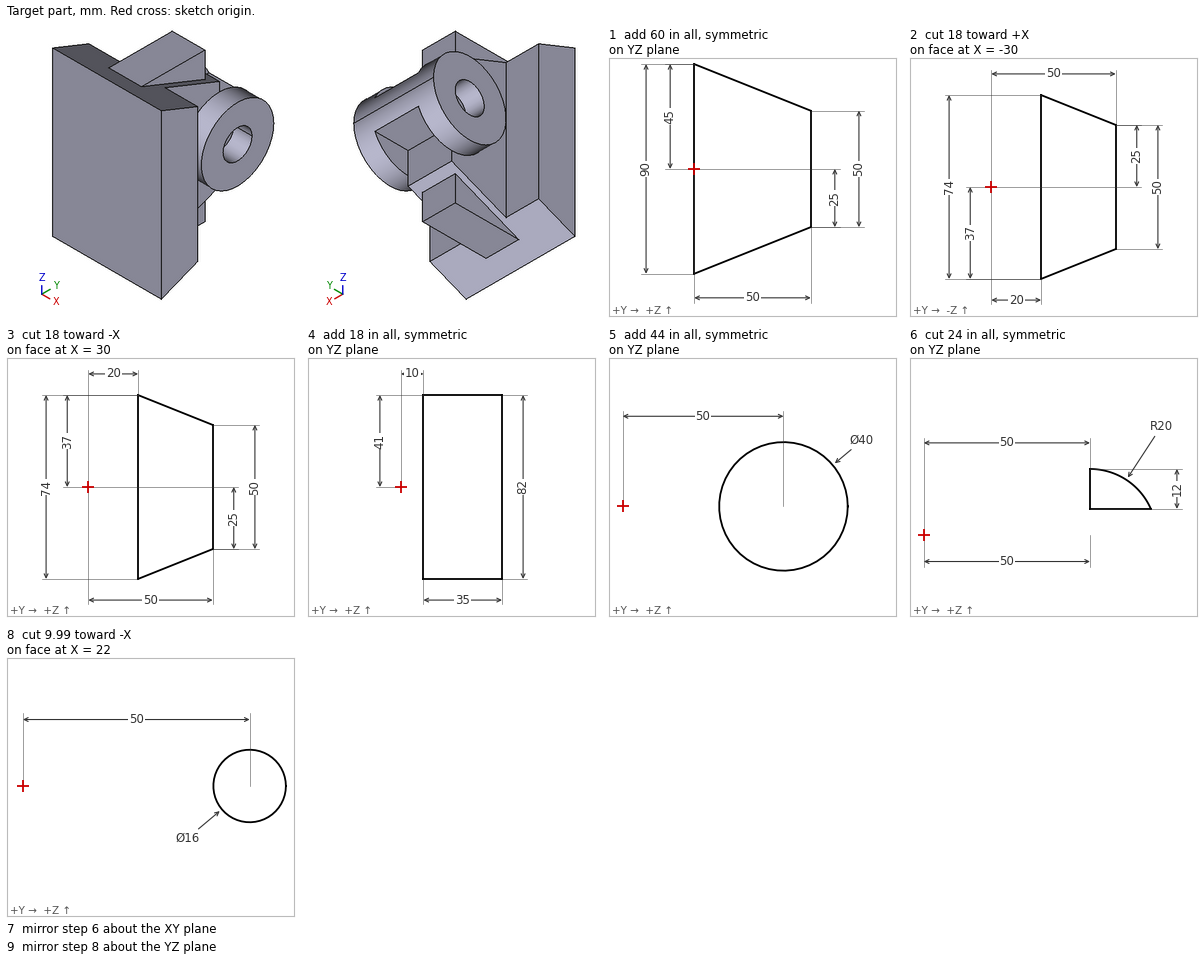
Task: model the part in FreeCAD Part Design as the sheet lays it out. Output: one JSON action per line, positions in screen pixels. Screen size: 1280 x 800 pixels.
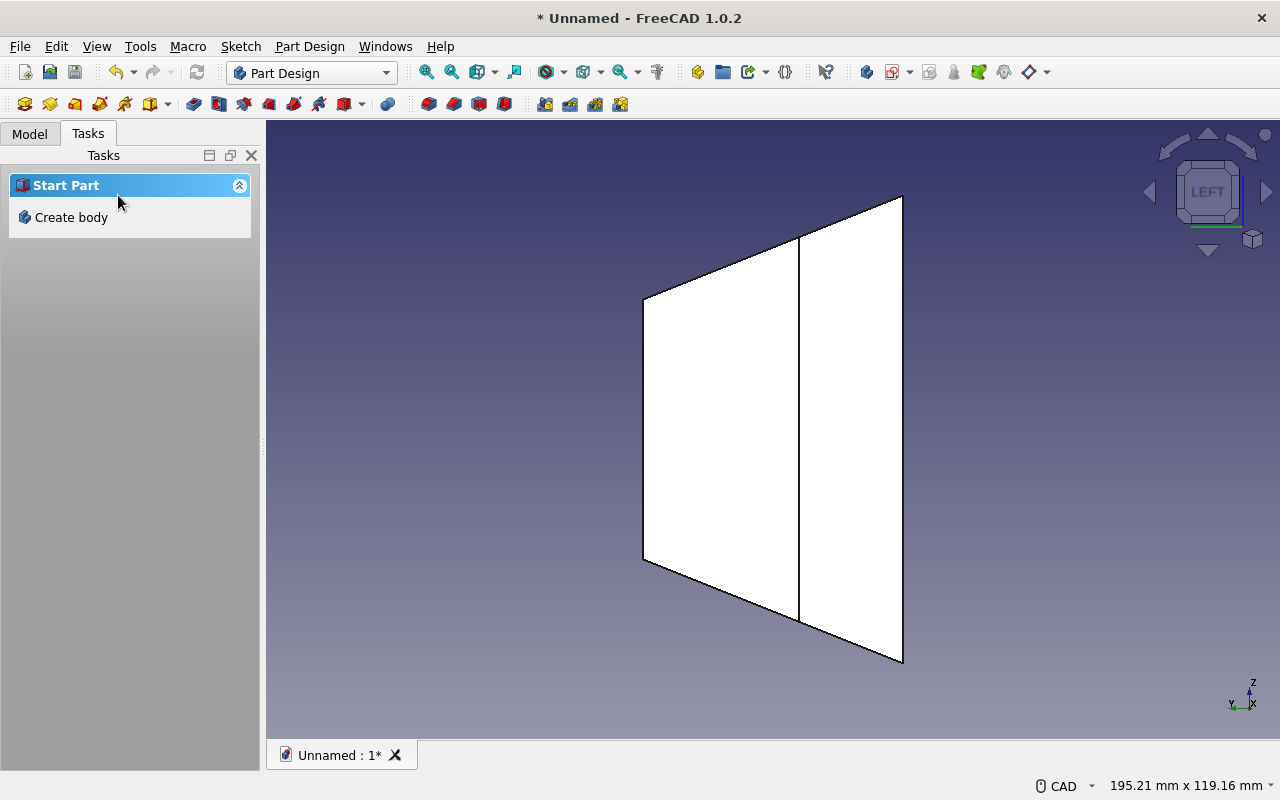
{"action": "key", "text": "0"}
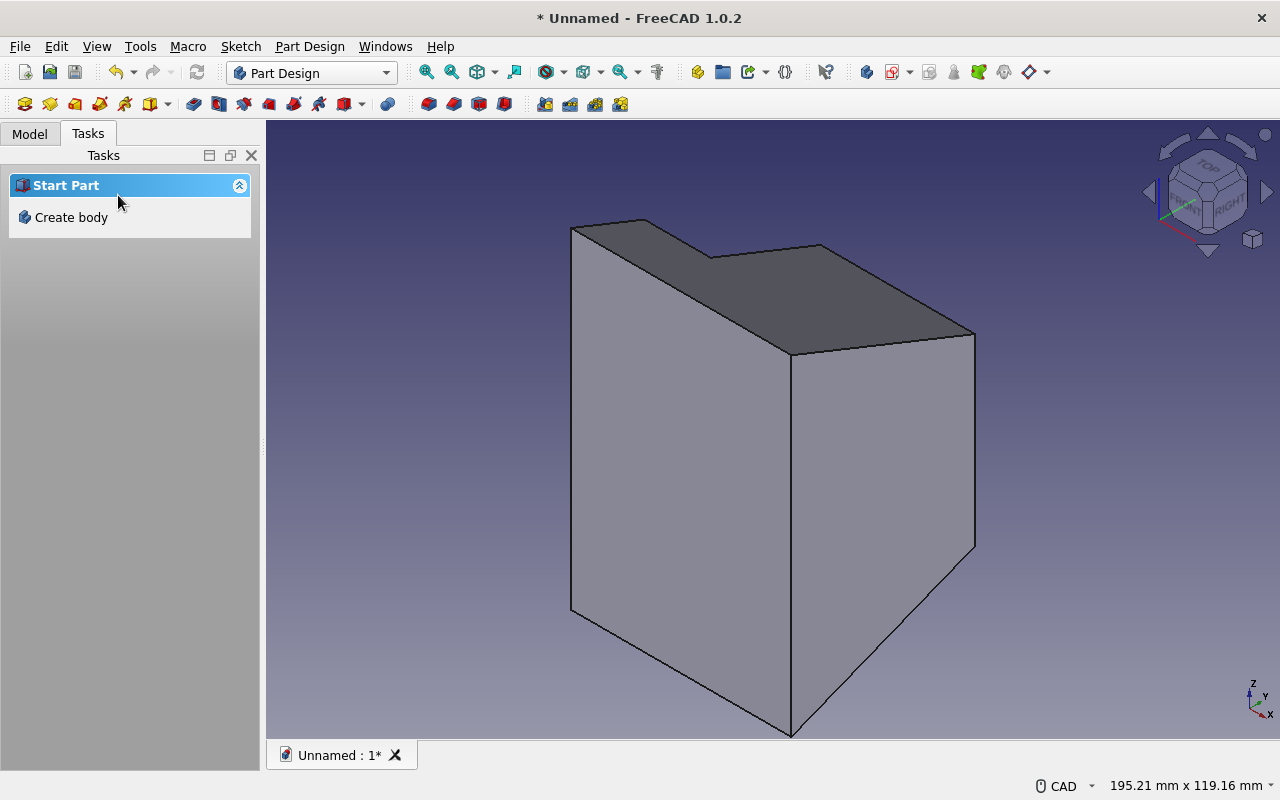
{"action": "left_click", "coordinate": [883, 492]}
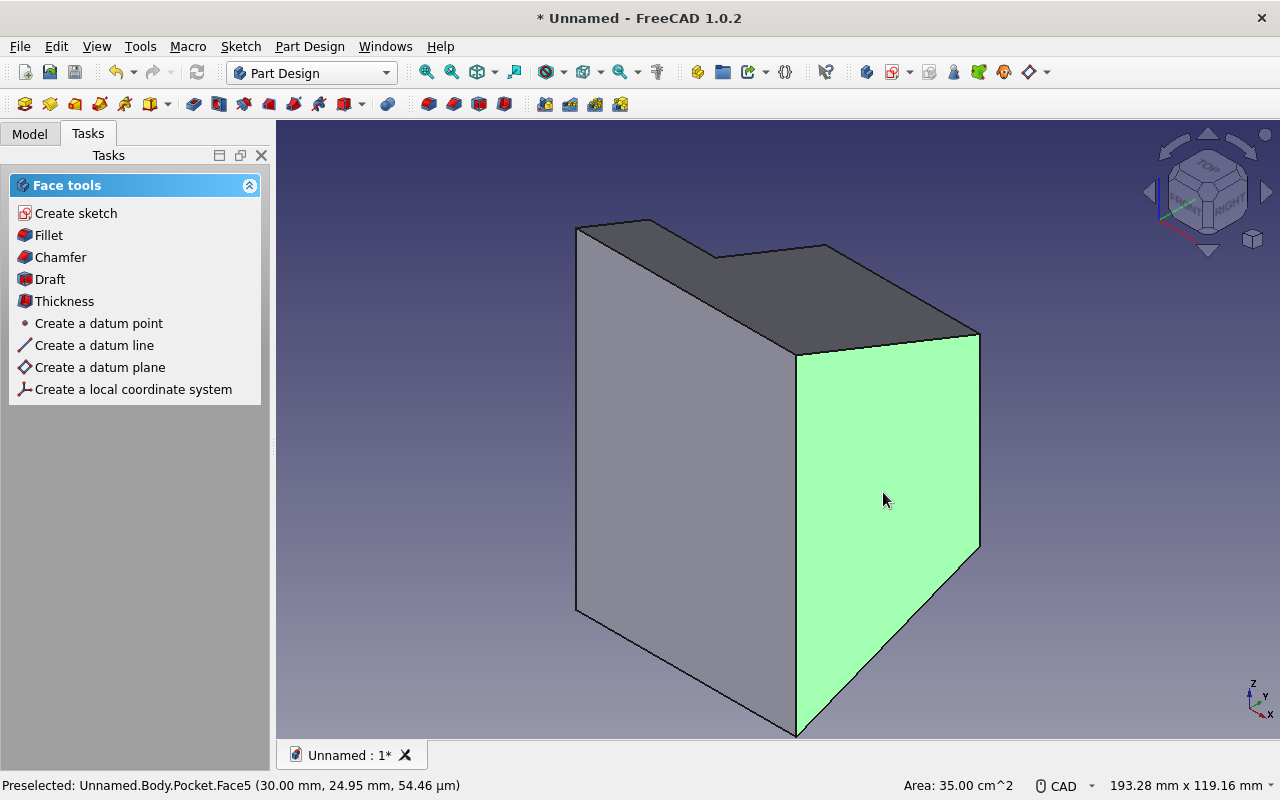
{"action": "left_click", "coordinate": [892, 72]}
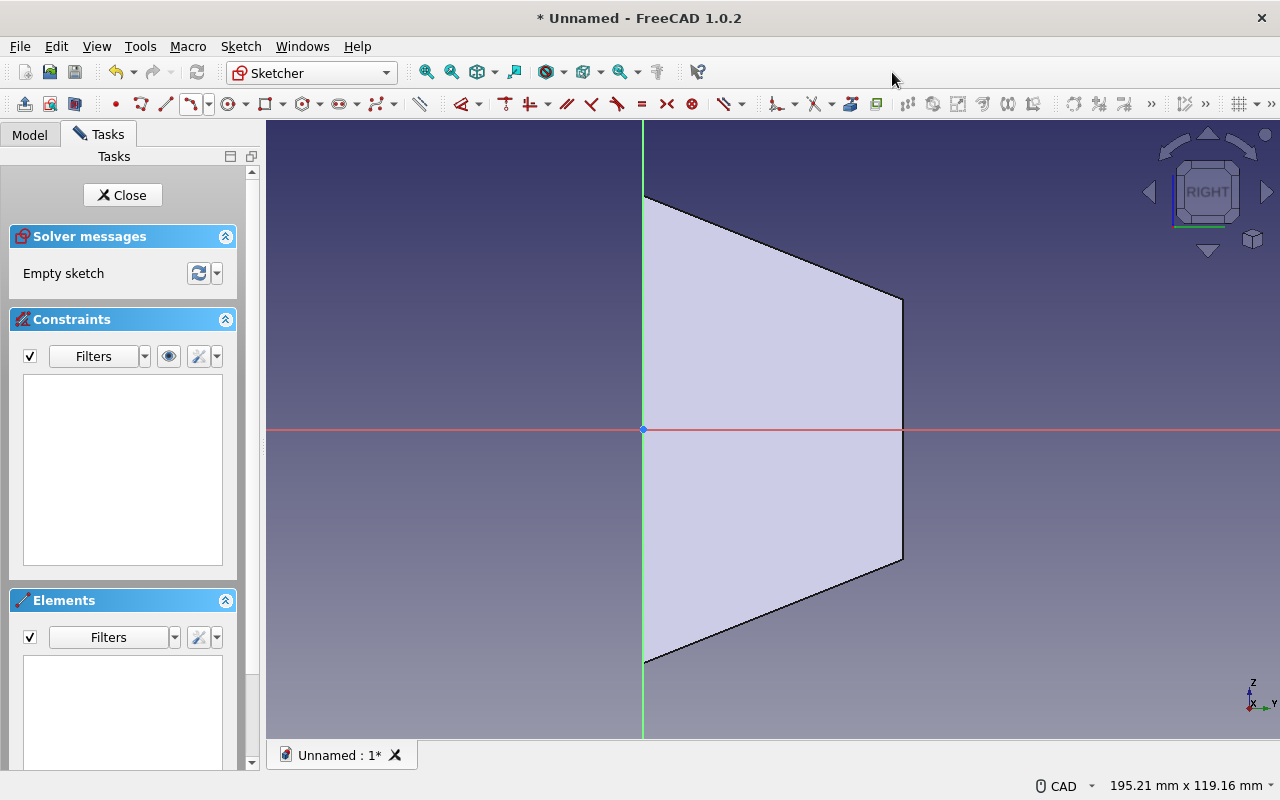
{"action": "left_click", "coordinate": [141, 104]}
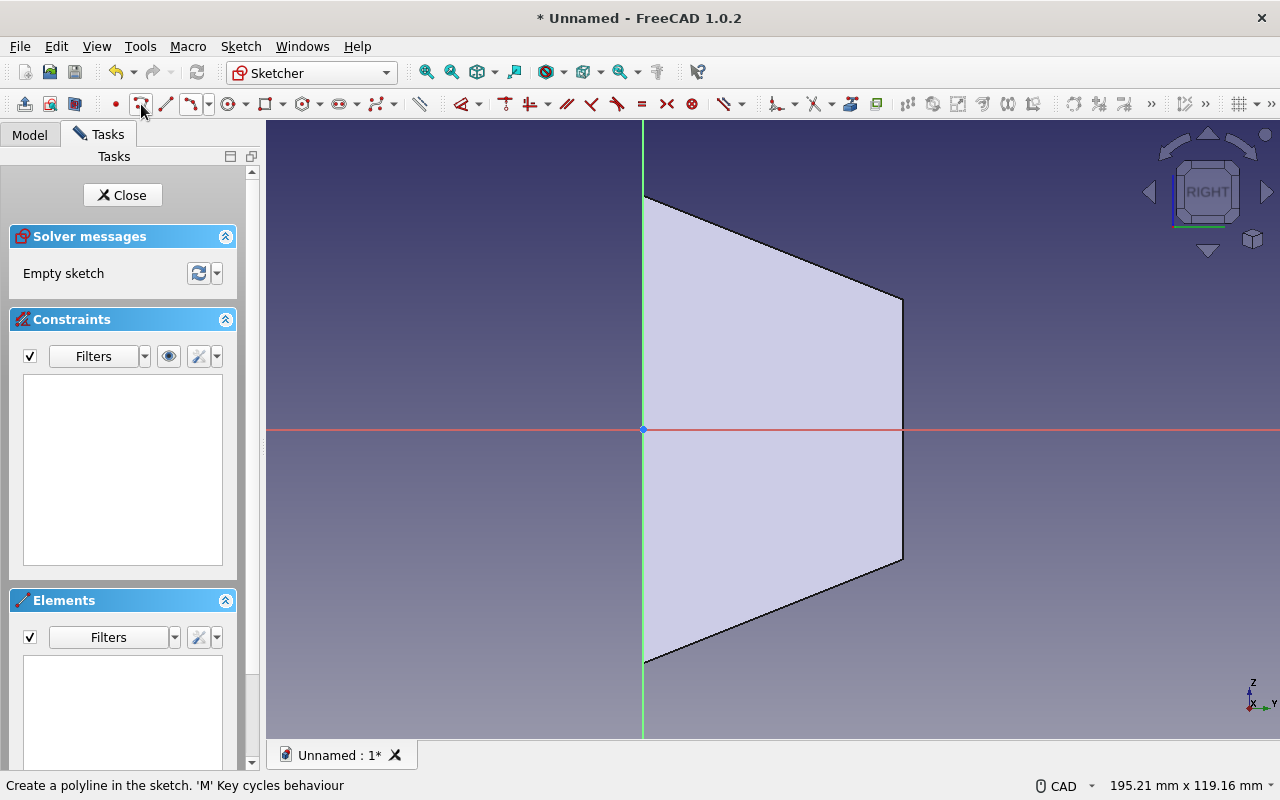
{"action": "left_click", "coordinate": [747, 237]}
{"action": "left_click", "coordinate": [747, 622]}
{"action": "left_click", "coordinate": [903, 559]}
{"action": "left_click", "coordinate": [903, 300]}
{"action": "left_click", "coordinate": [747, 238]}
{"action": "key", "text": "Escape"}
{"action": "key", "text": "Escape"}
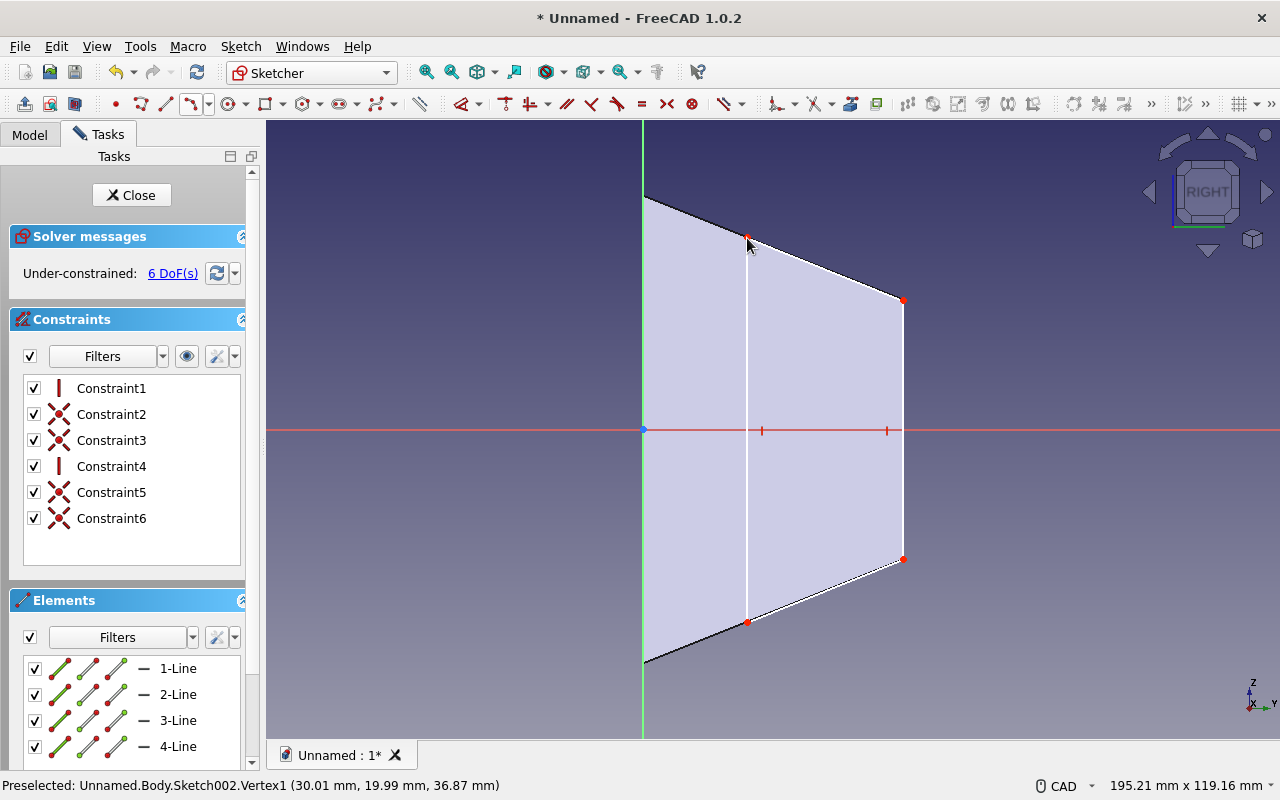
{"action": "left_click", "coordinate": [460, 104]}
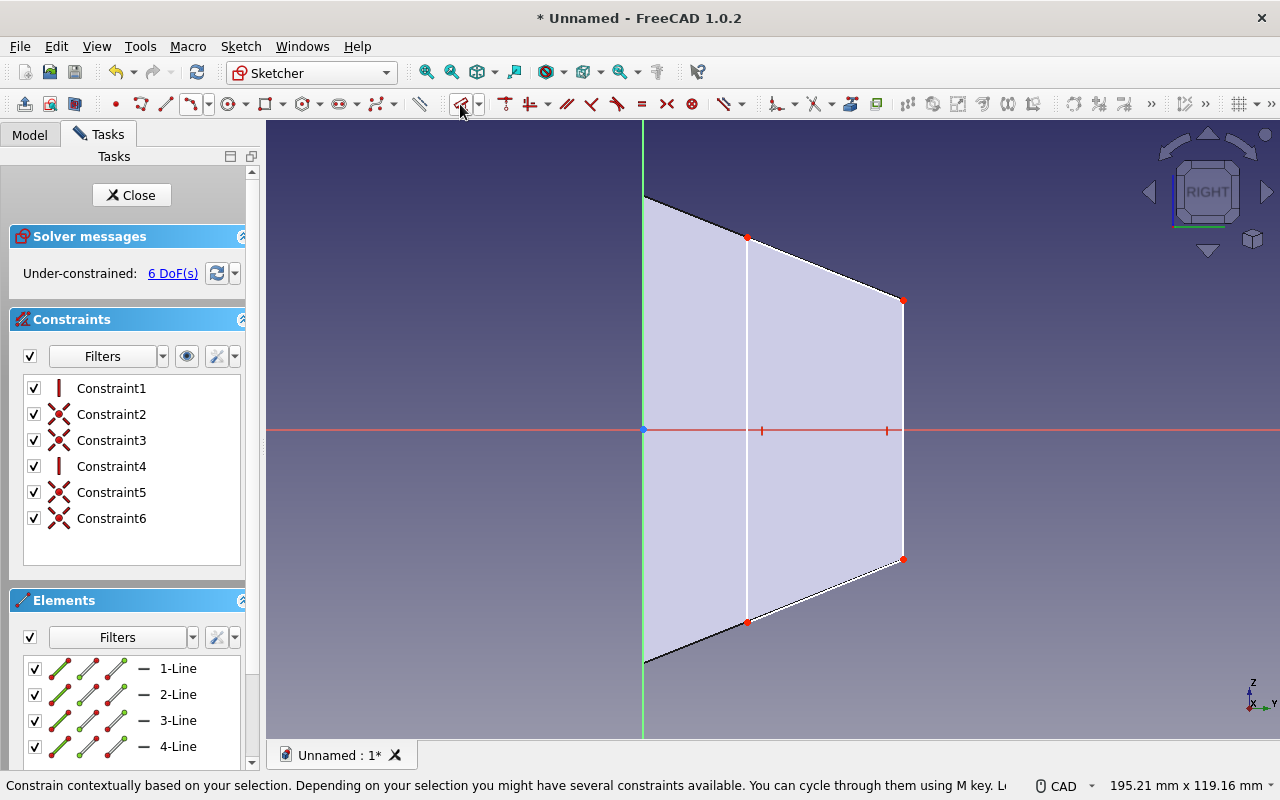
{"action": "left_click", "coordinate": [747, 353]}
{"action": "left_click", "coordinate": [713, 342]}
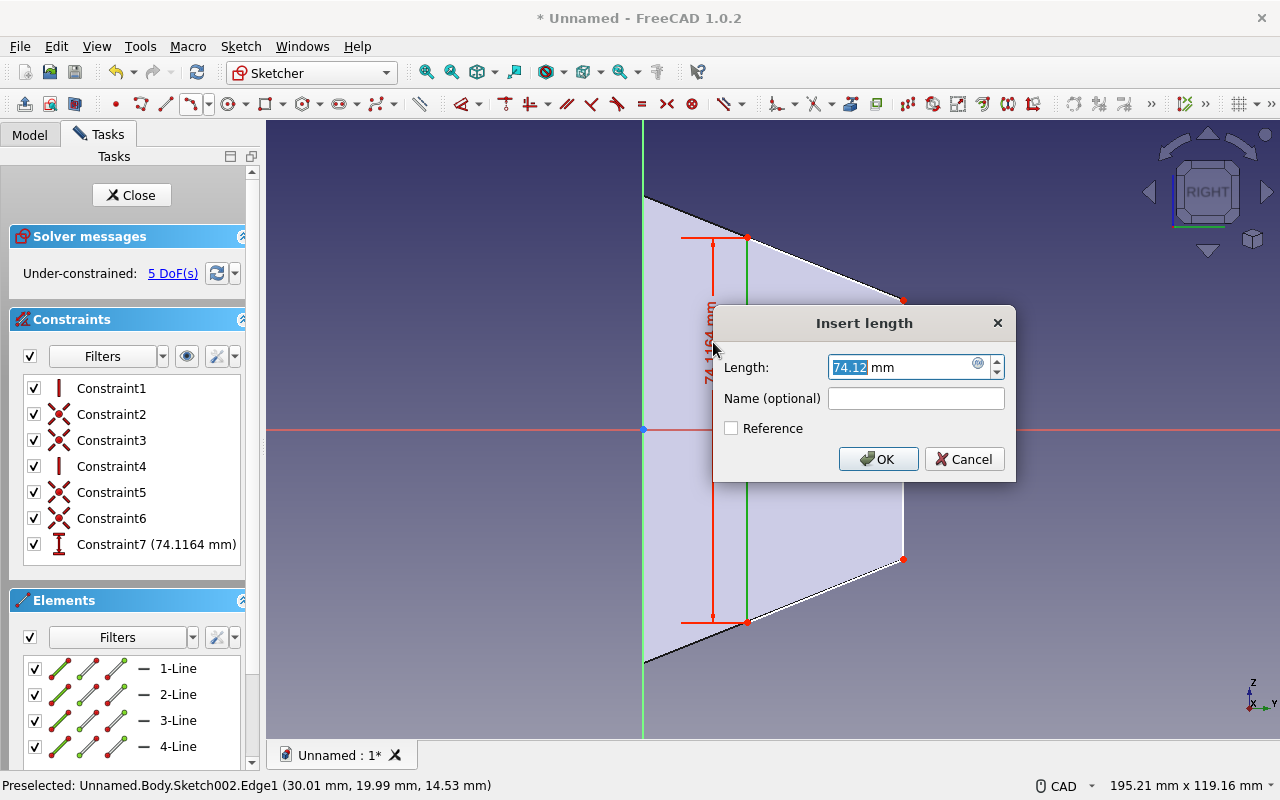
{"action": "type", "text": "74"}
{"action": "key", "text": "Return"}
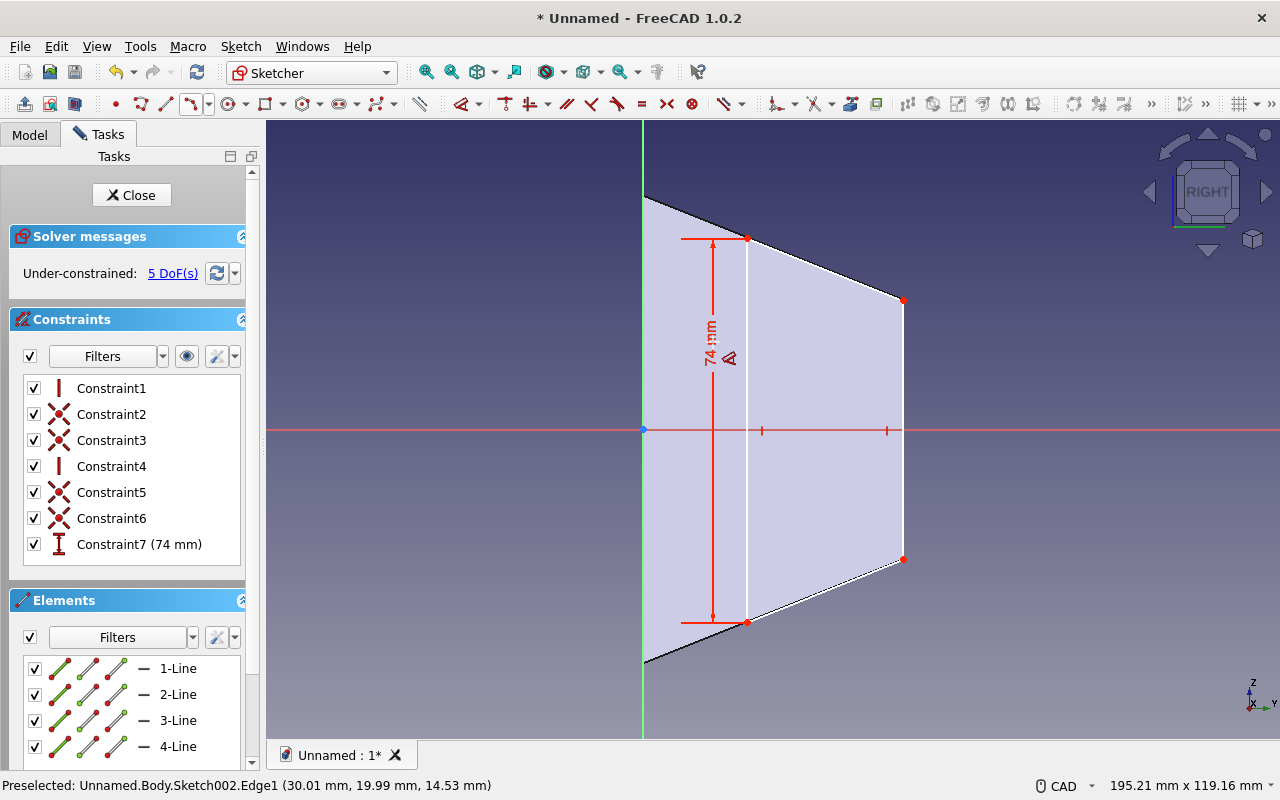
{"action": "left_click", "coordinate": [903, 482]}
{"action": "left_click", "coordinate": [937, 371]}